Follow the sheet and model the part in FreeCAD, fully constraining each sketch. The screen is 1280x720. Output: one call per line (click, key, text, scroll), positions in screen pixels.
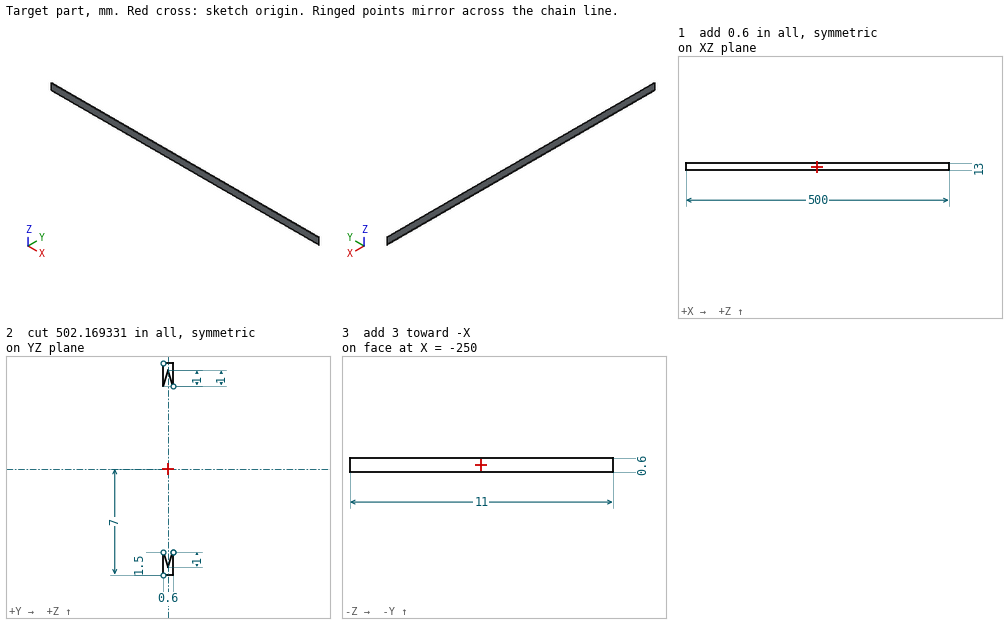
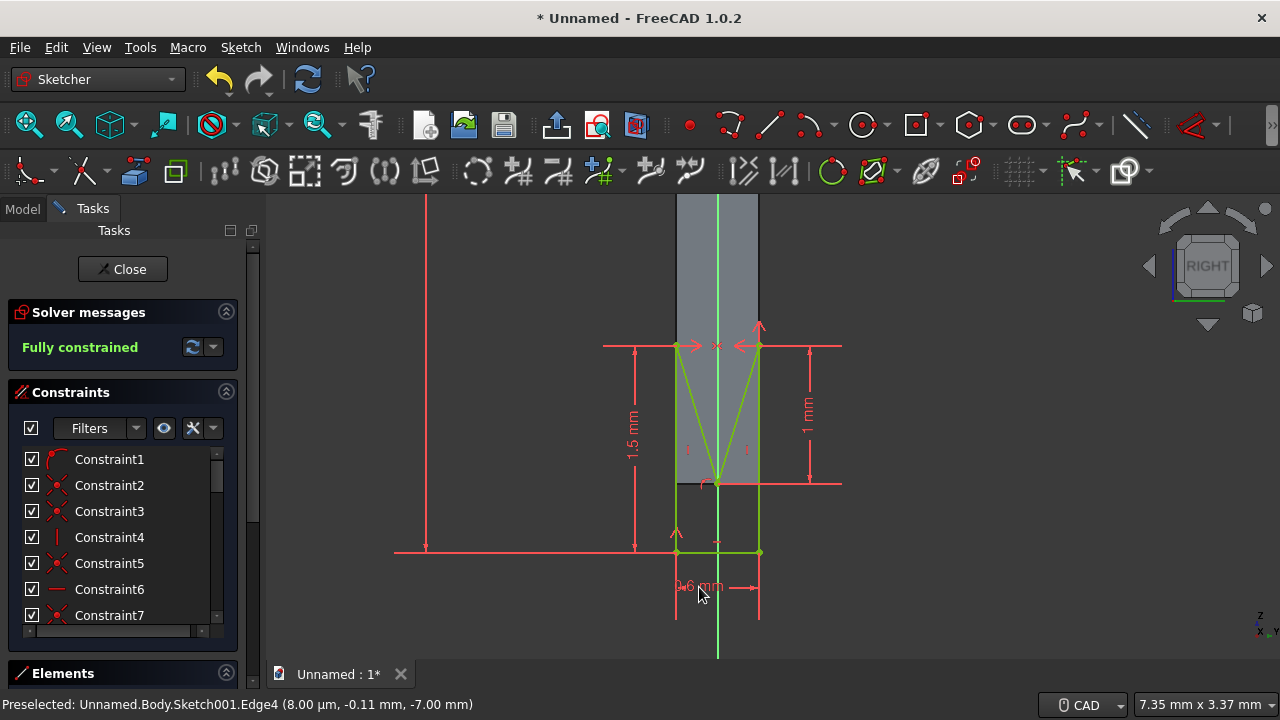
click(123, 269)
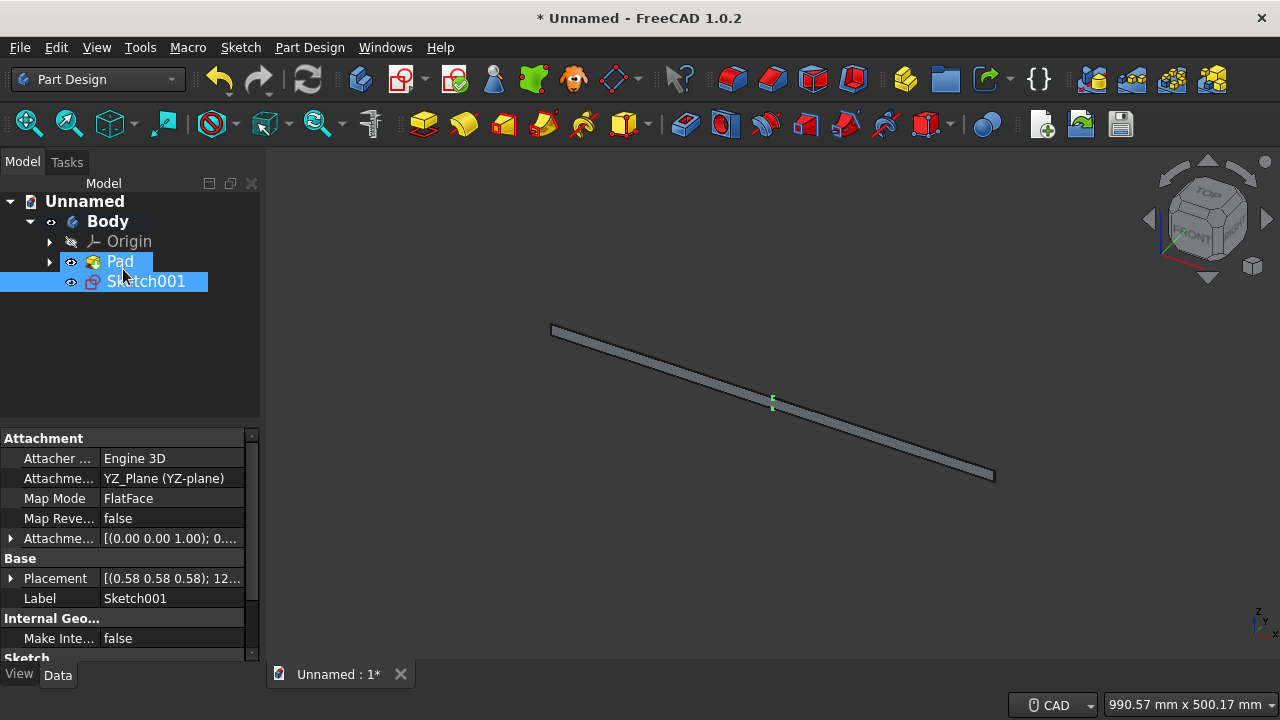
click(686, 124)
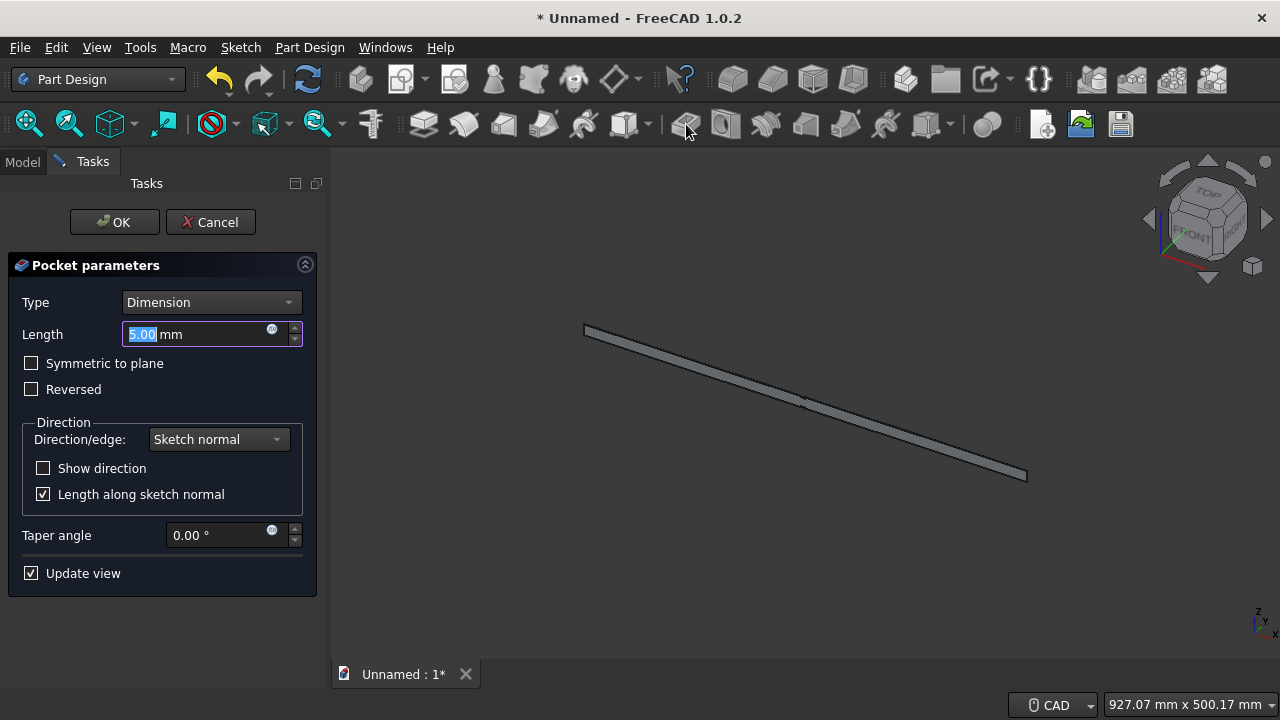
text(502.169331)
key(Tab)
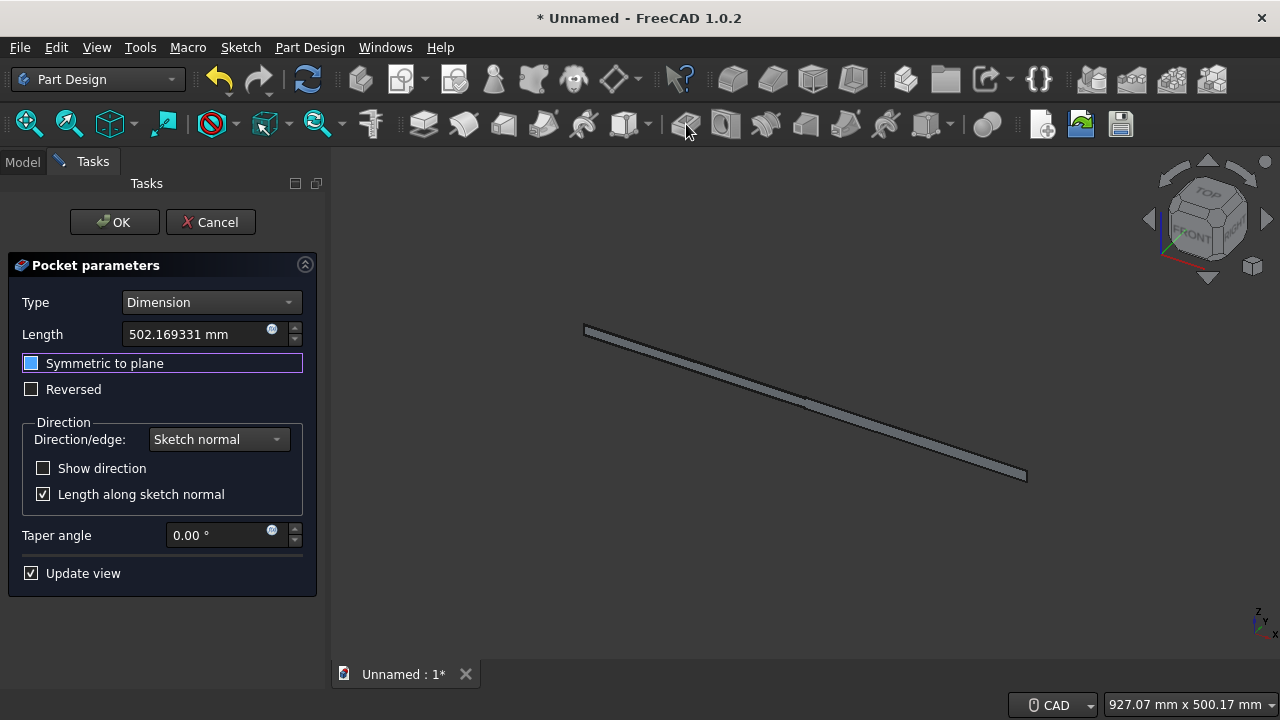
click(30, 363)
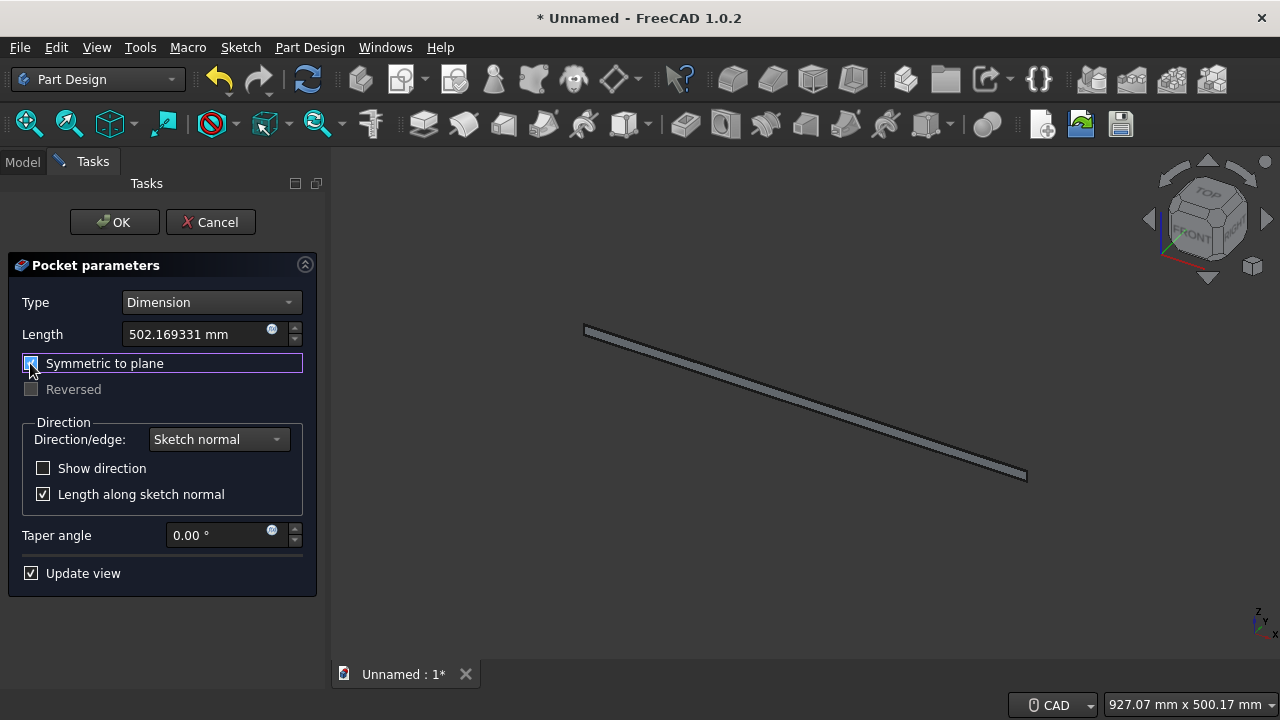
click(115, 222)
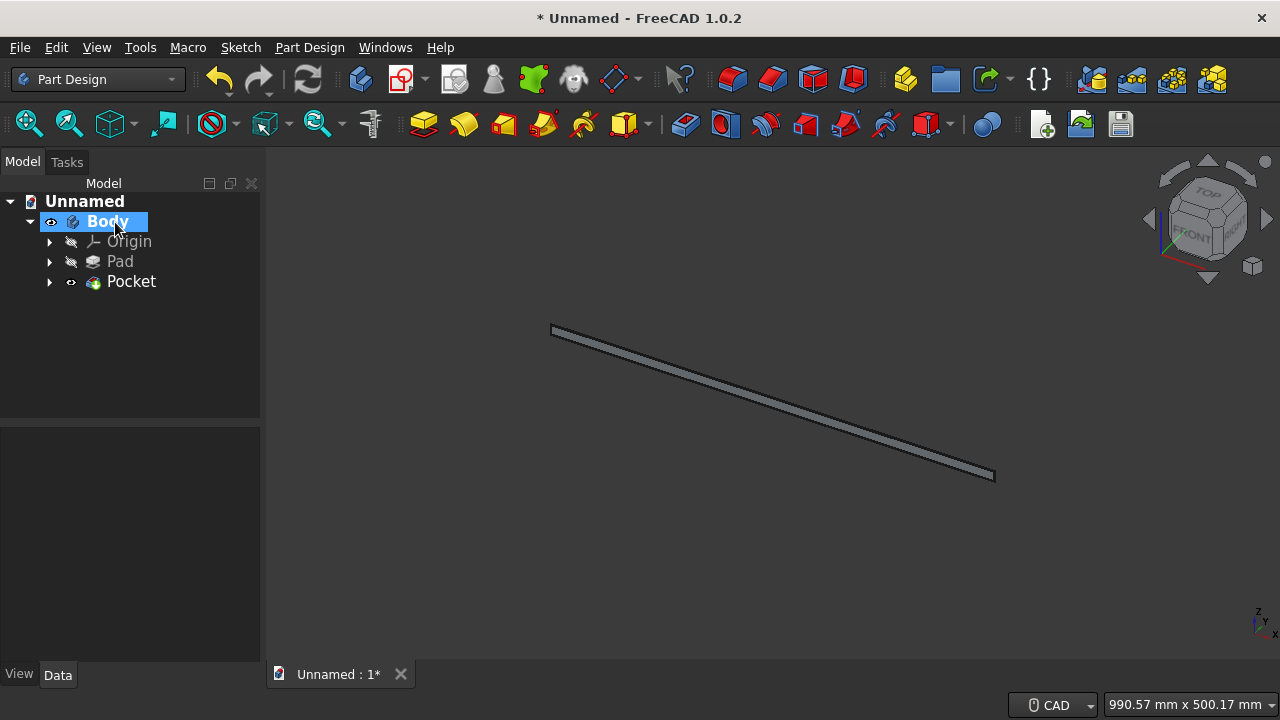
click(30, 124)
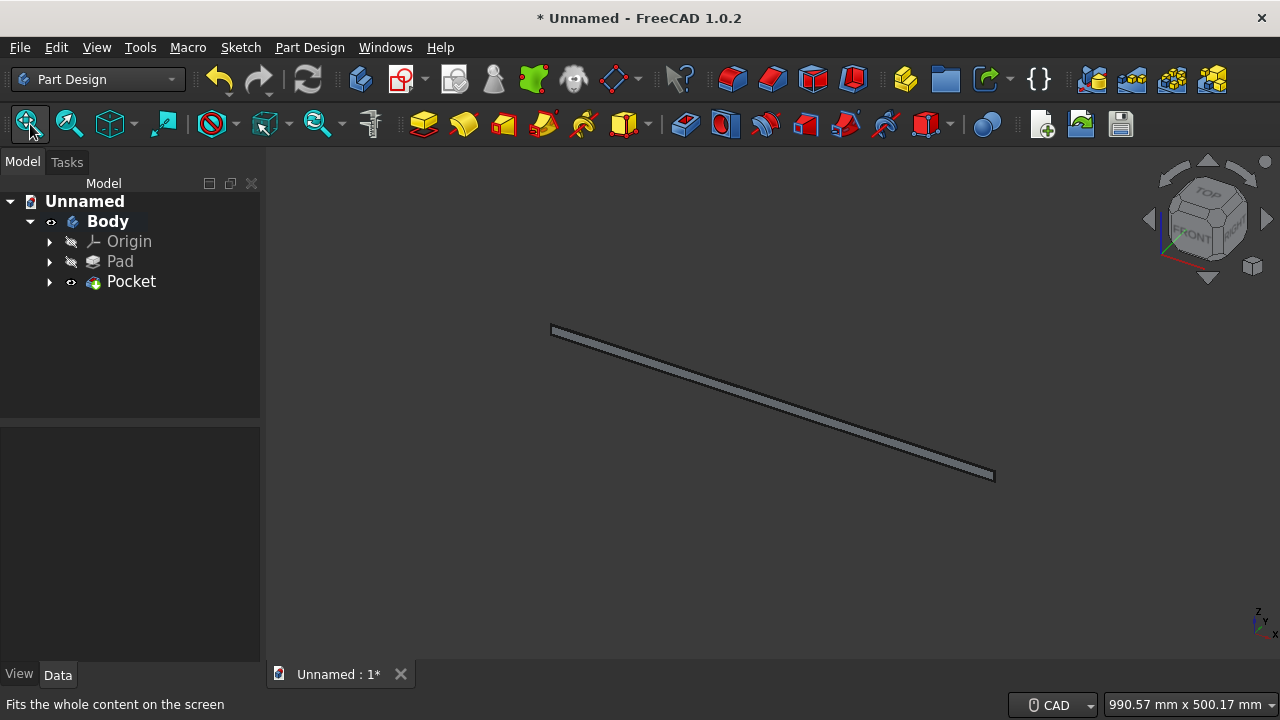
key(6)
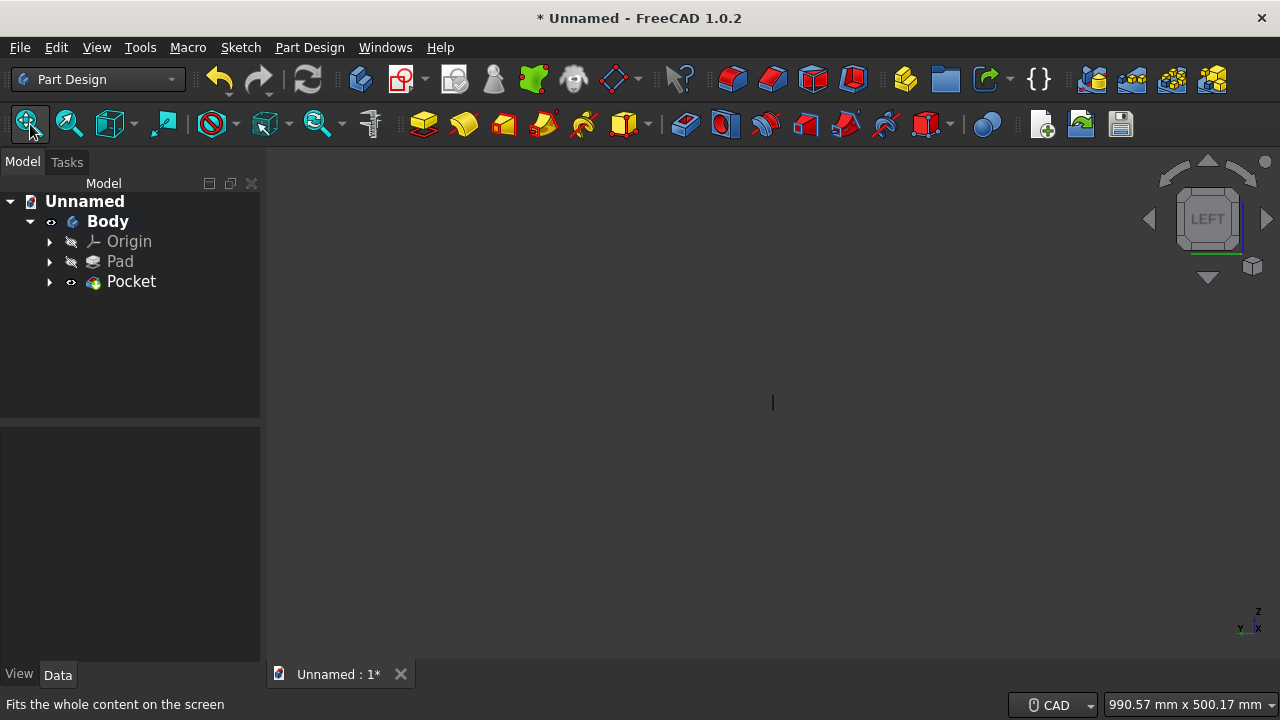
click(30, 124)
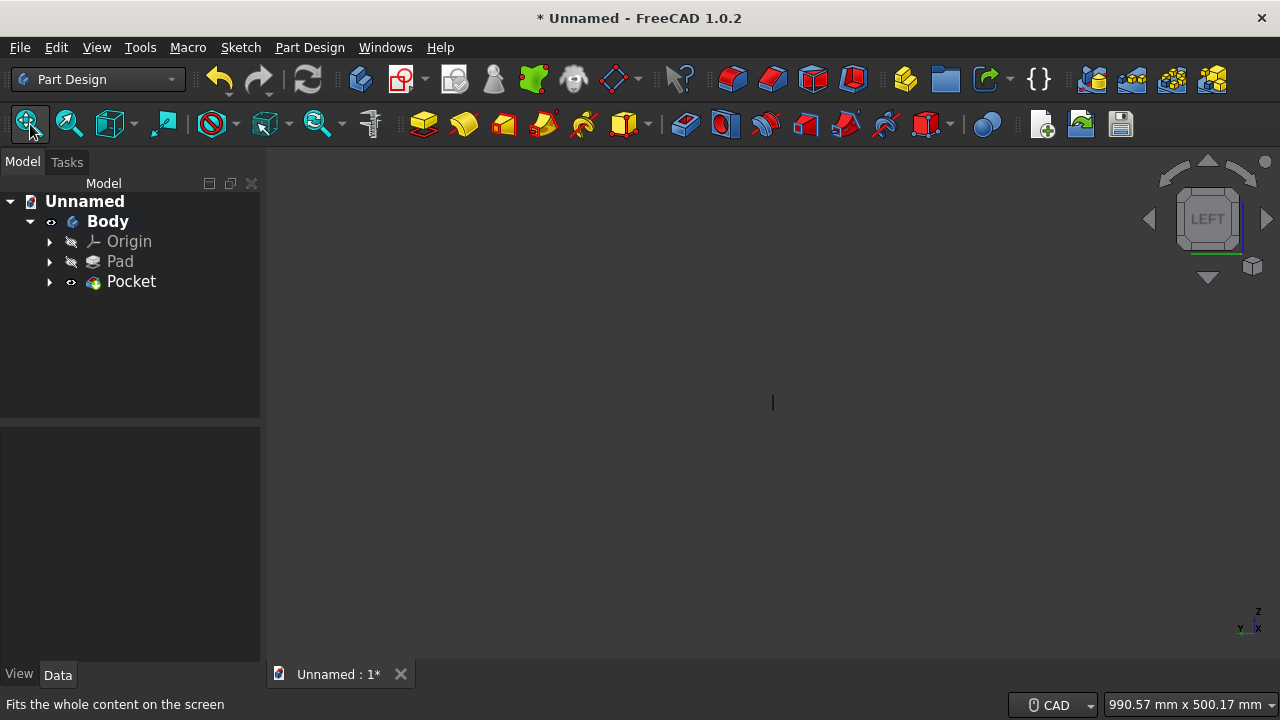
scroll(773, 398, up, 15)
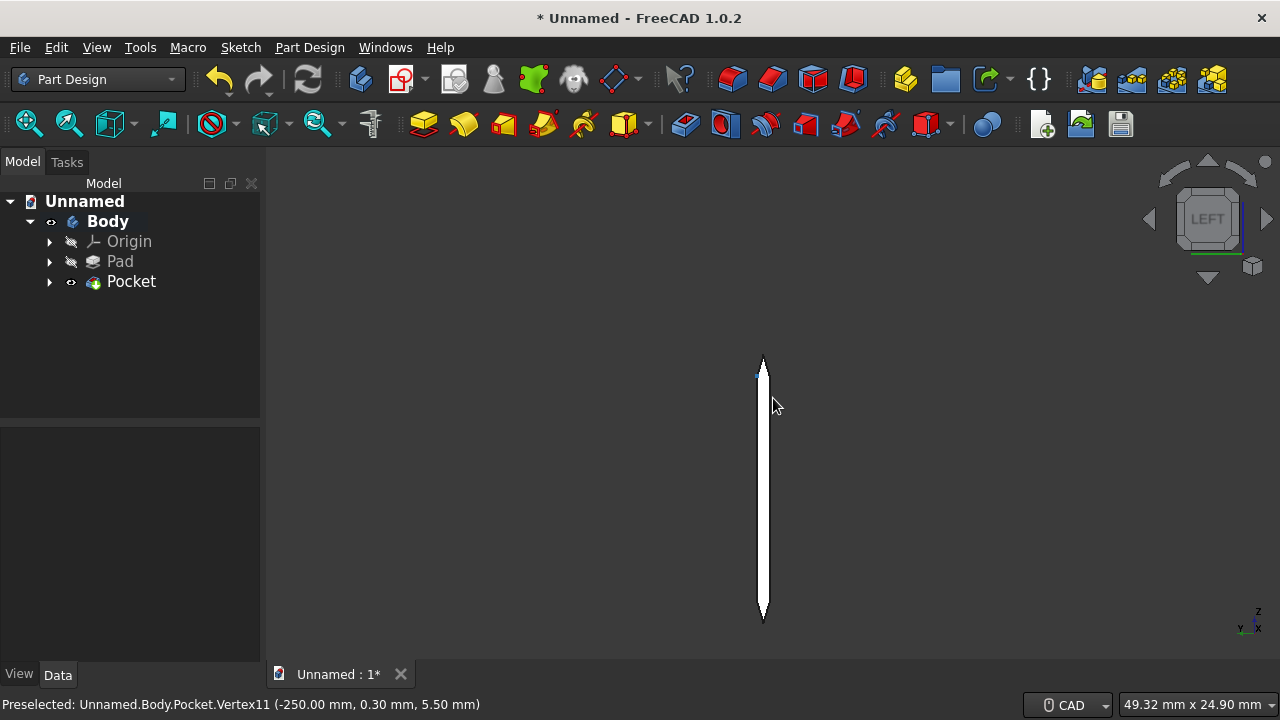
scroll(763, 412, up, 4)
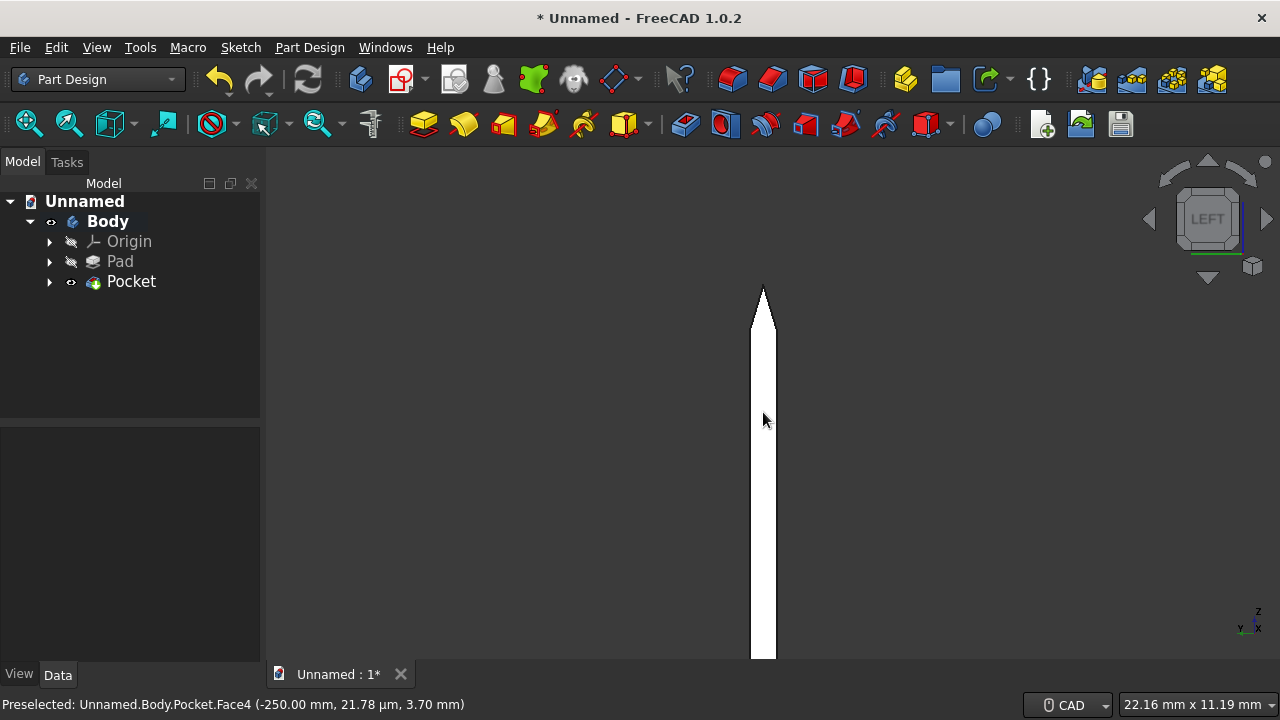
click(763, 412)